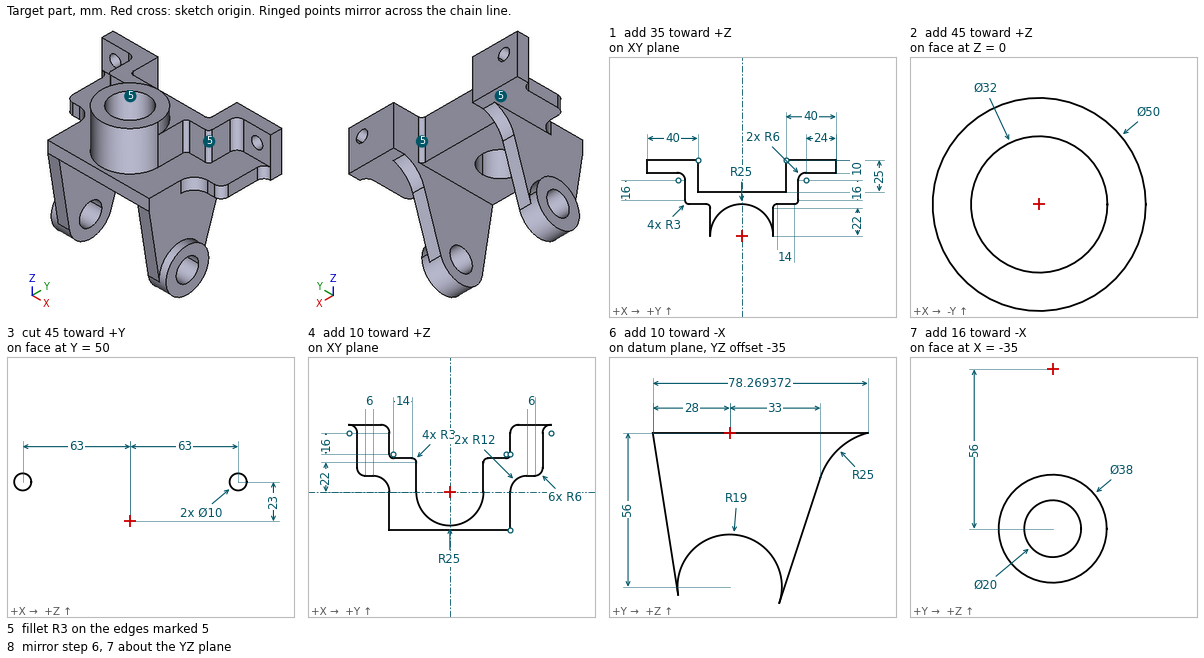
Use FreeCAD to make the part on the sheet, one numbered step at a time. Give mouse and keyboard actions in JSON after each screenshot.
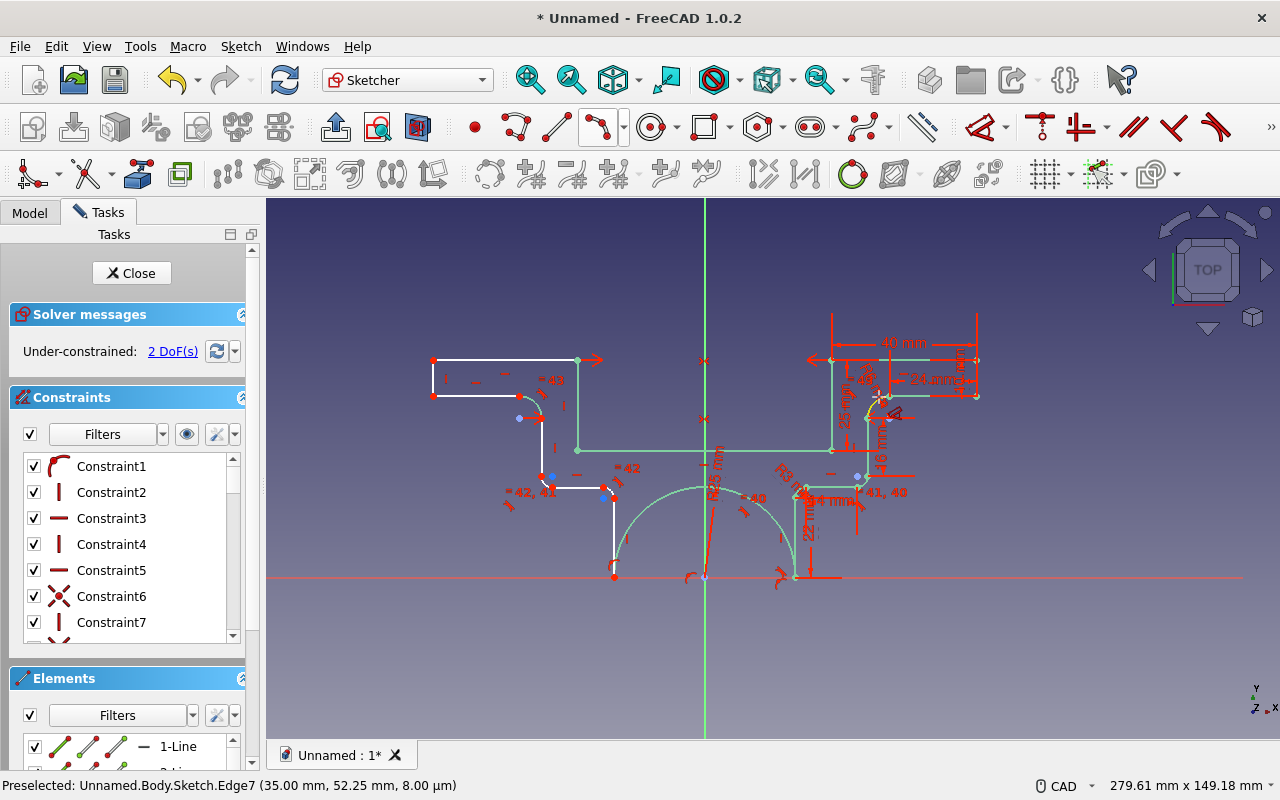
{"action": "left_click", "coordinate": [534, 360]}
{"action": "left_click", "coordinate": [506, 326]}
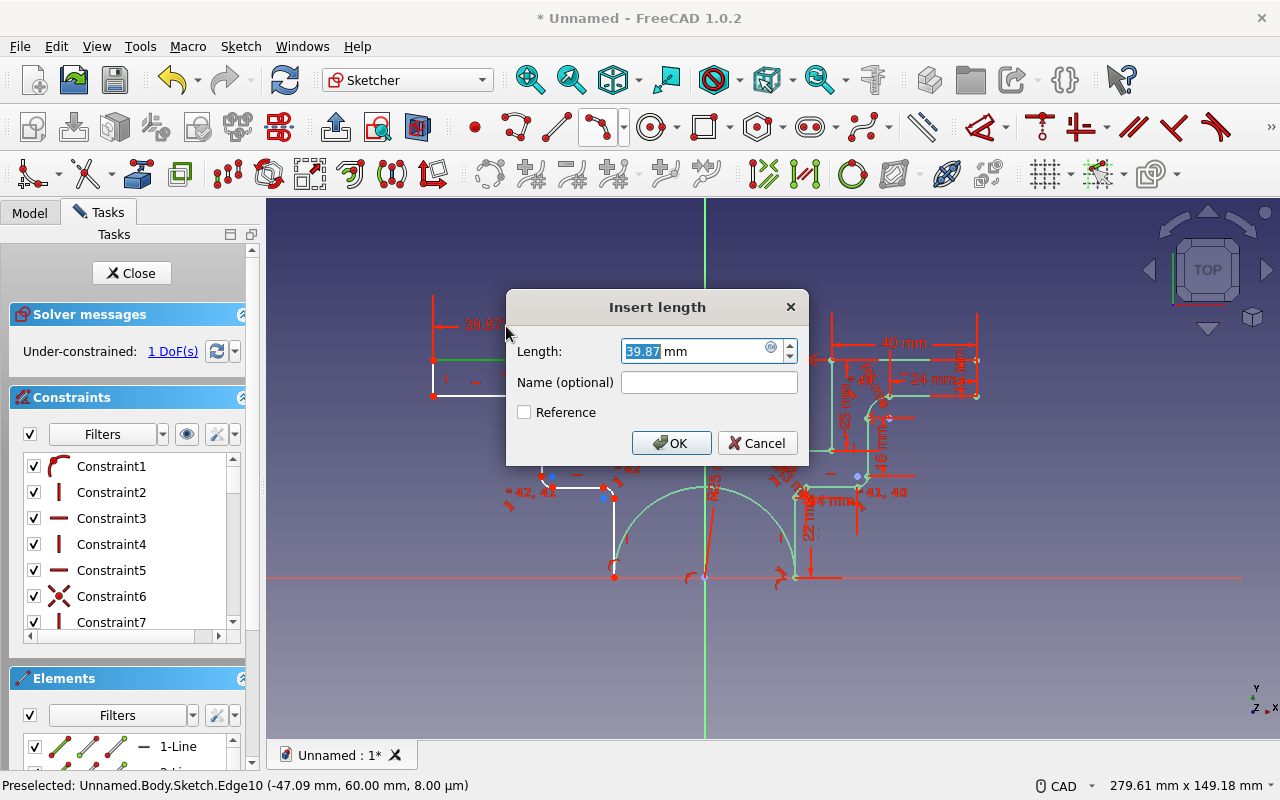
{"action": "type", "text": "40"}
{"action": "key", "text": "Return"}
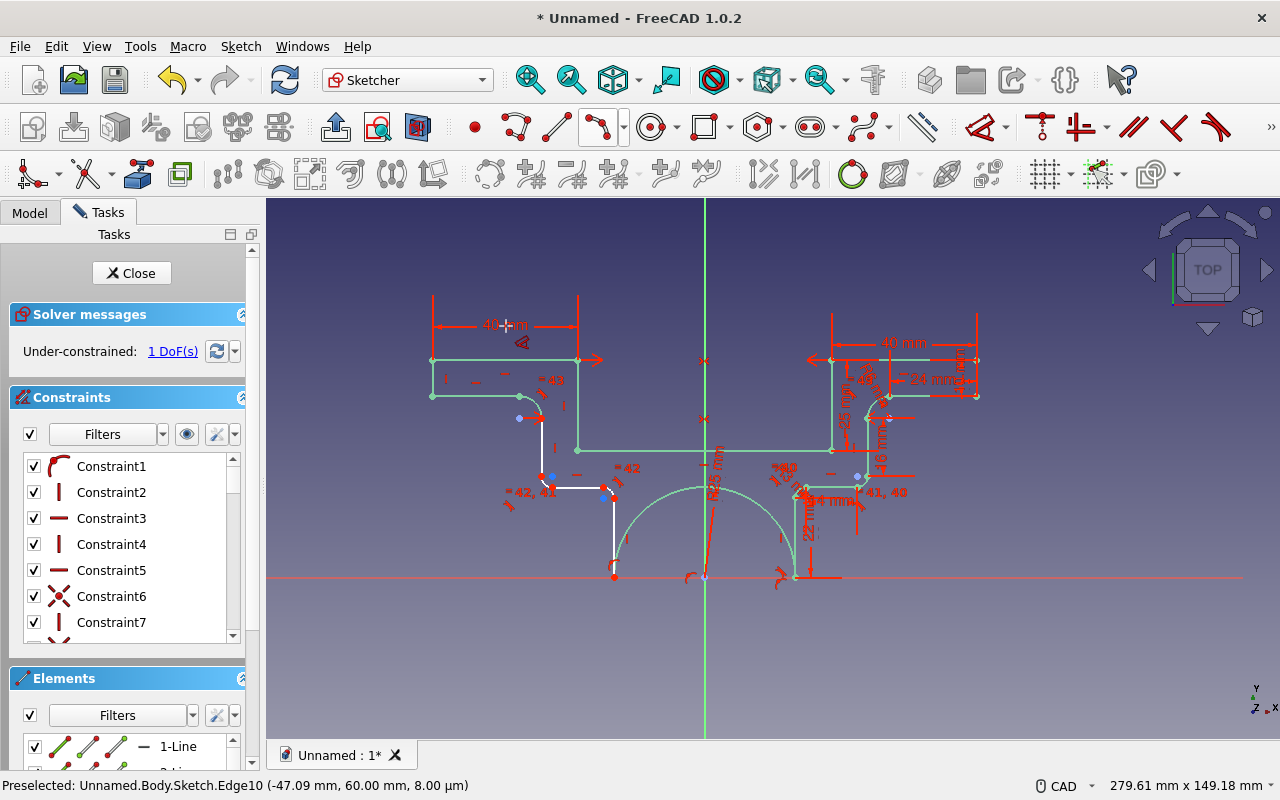
{"action": "left_click", "coordinate": [542, 436]}
{"action": "left_click", "coordinate": [508, 447]}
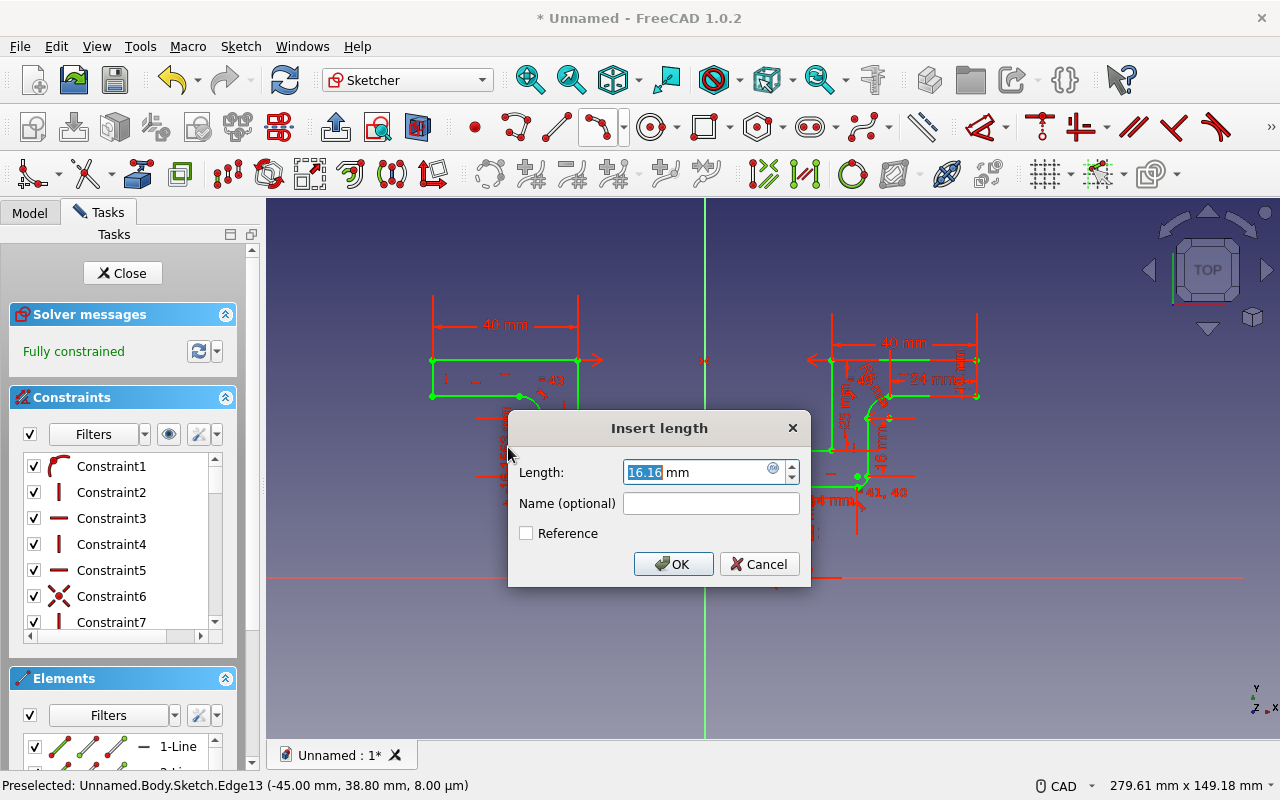
{"action": "type", "text": "16"}
{"action": "key", "text": "Return"}
{"action": "key", "text": "Escape"}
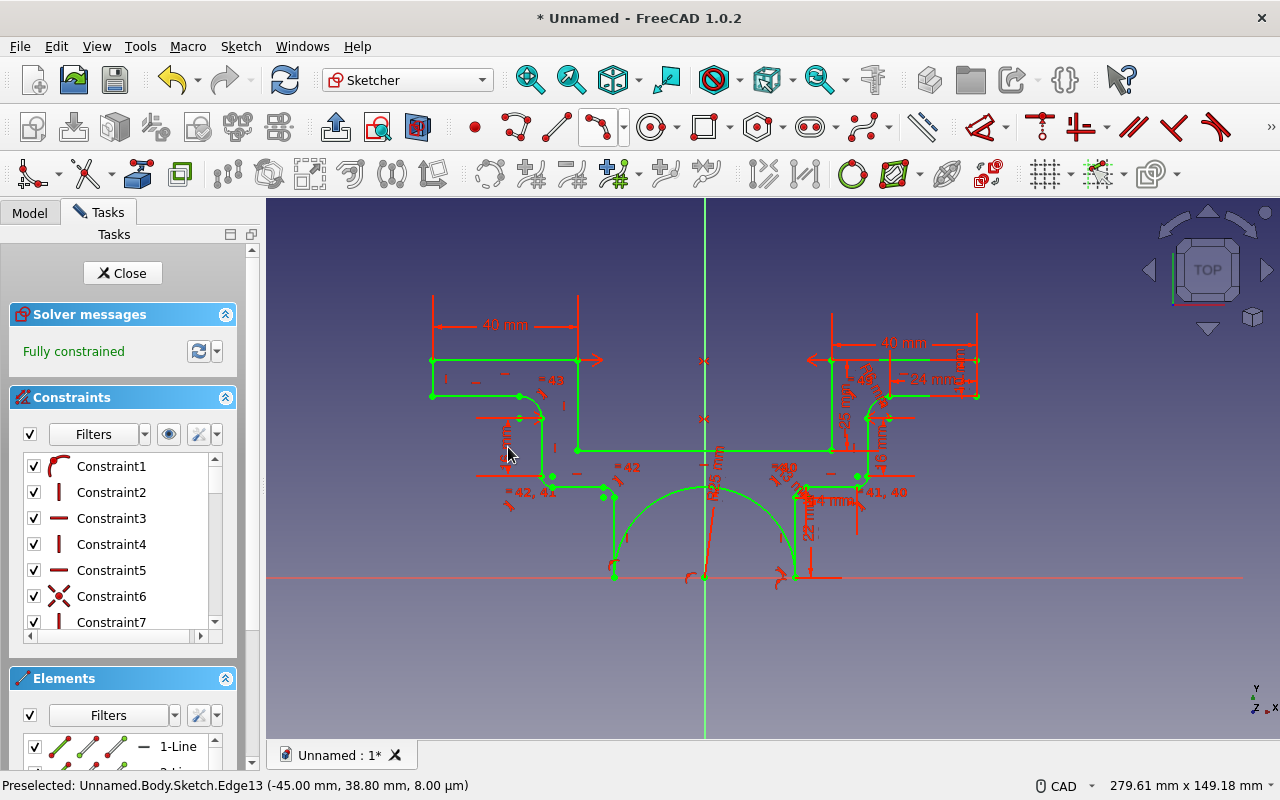
{"action": "left_click", "coordinate": [123, 273]}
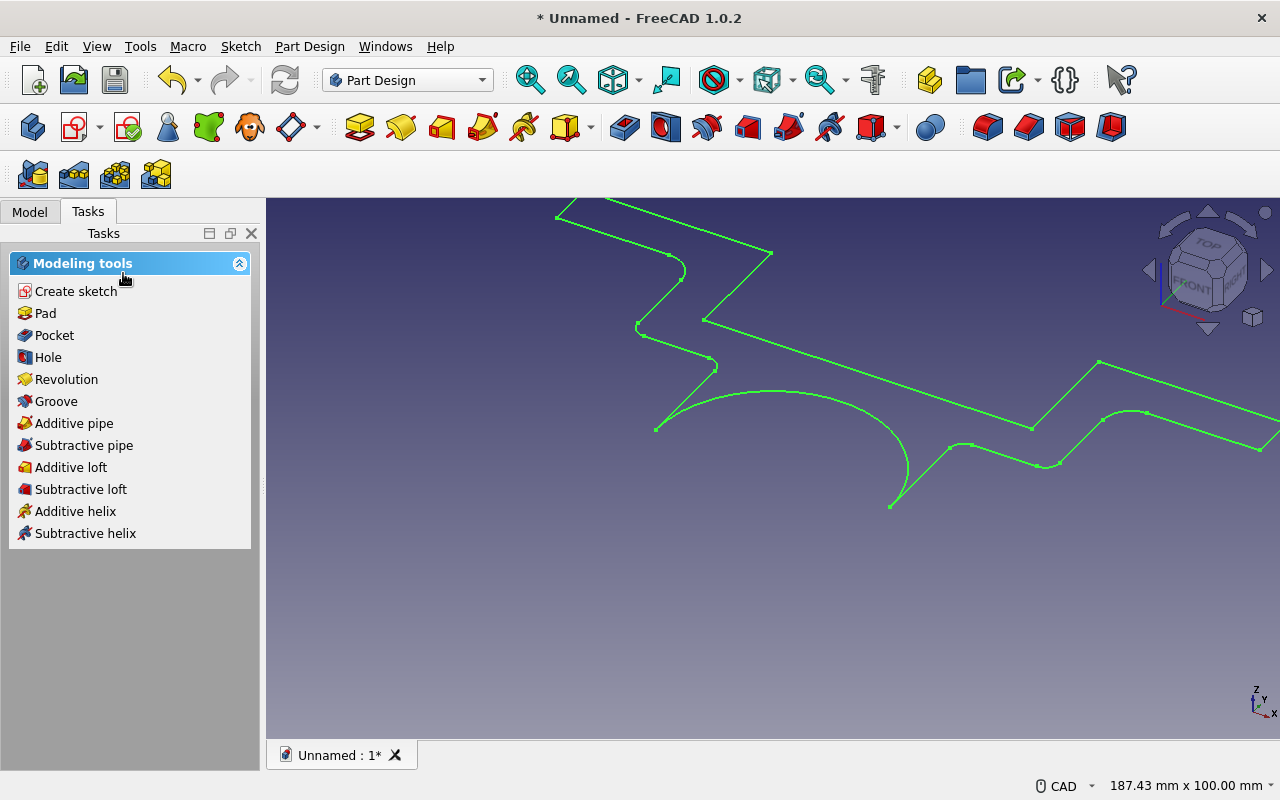
{"action": "left_click", "coordinate": [360, 128]}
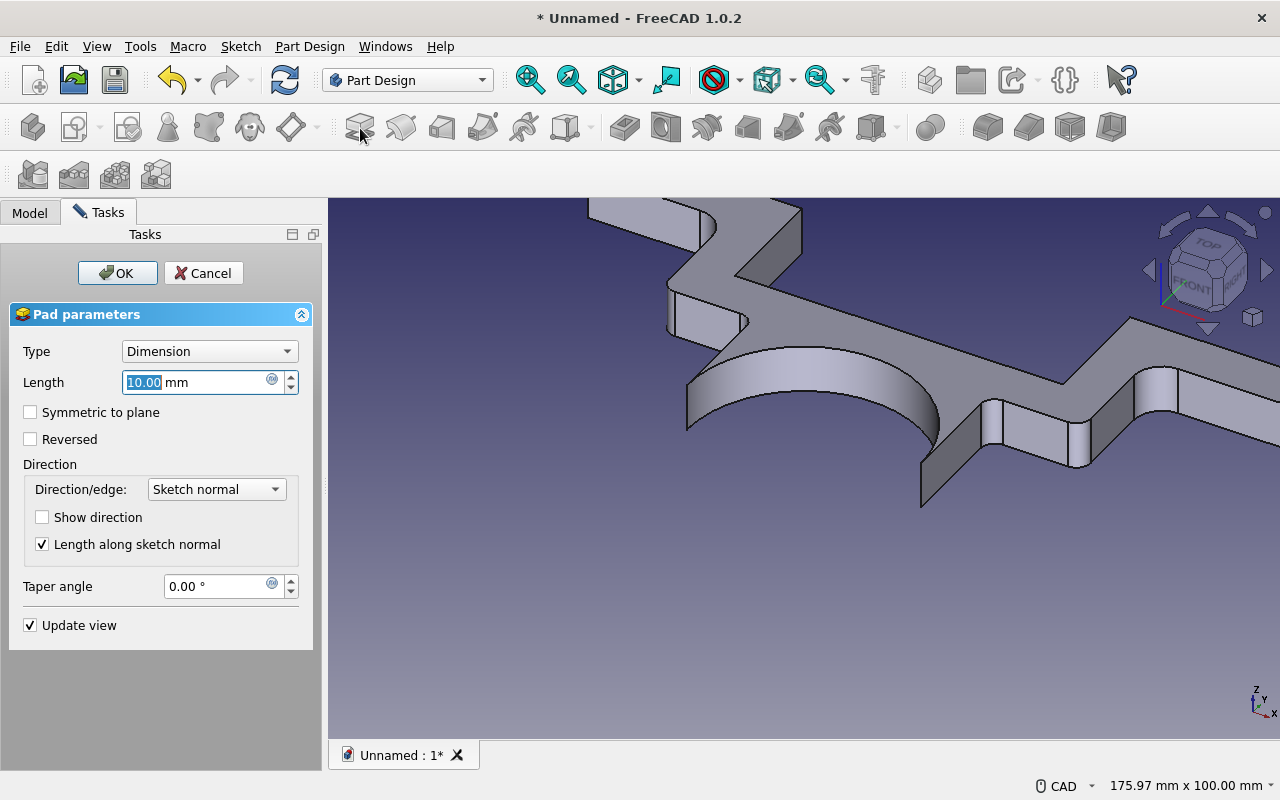
{"action": "type", "text": "35"}
{"action": "key", "text": "Tab"}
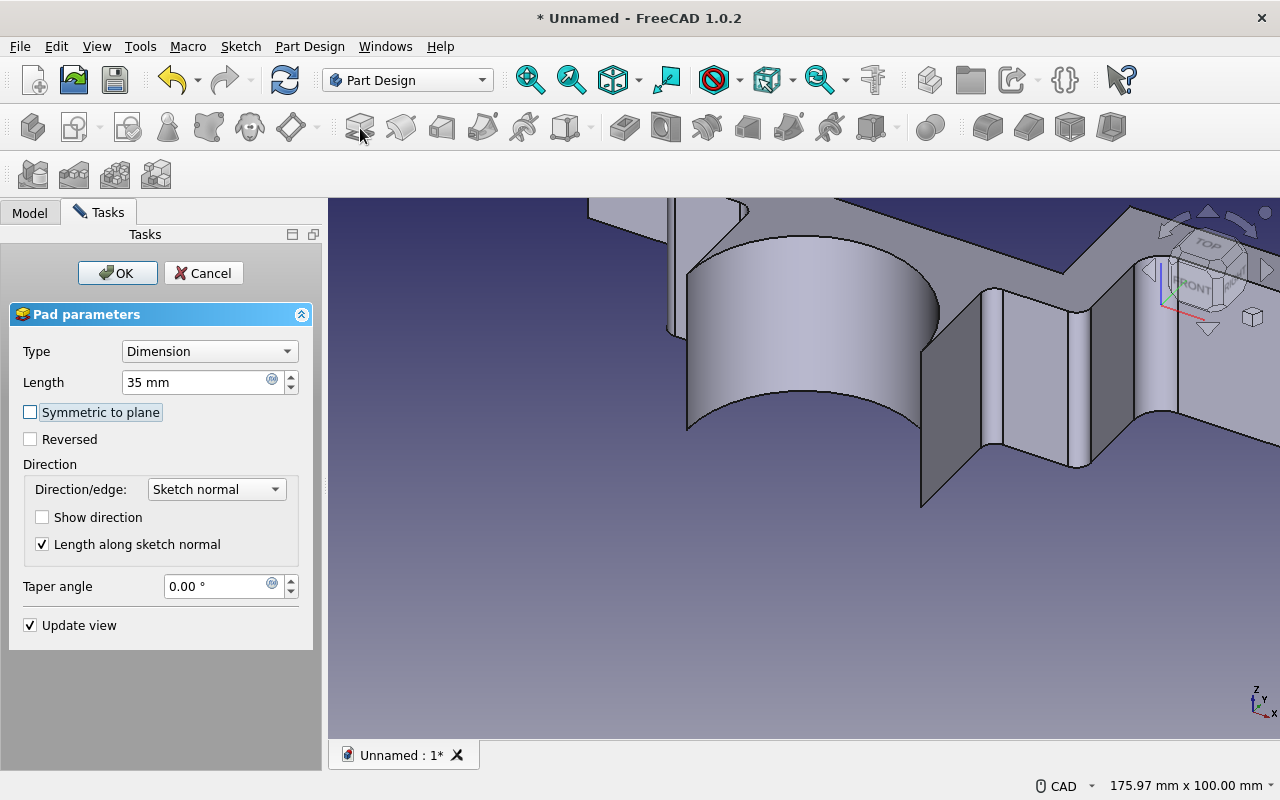
{"action": "left_click", "coordinate": [118, 273]}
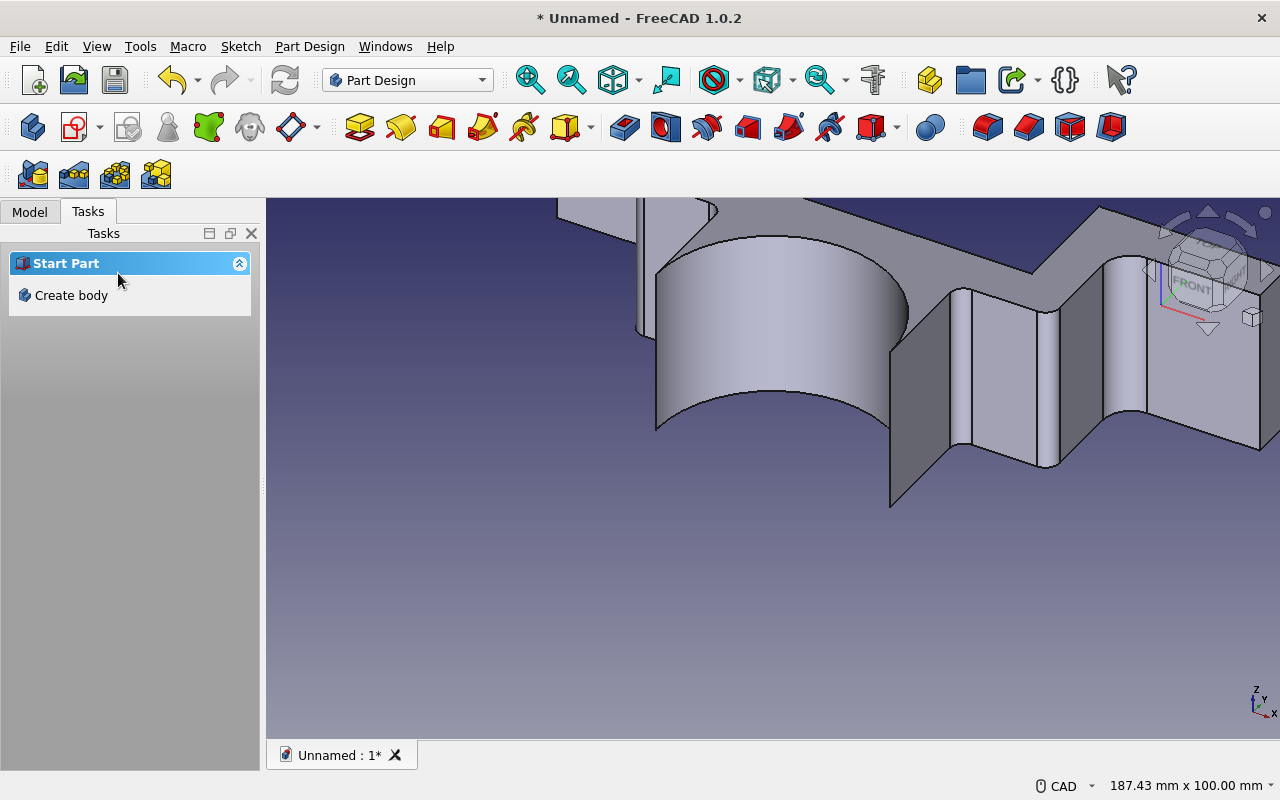
{"action": "left_click", "coordinate": [531, 80]}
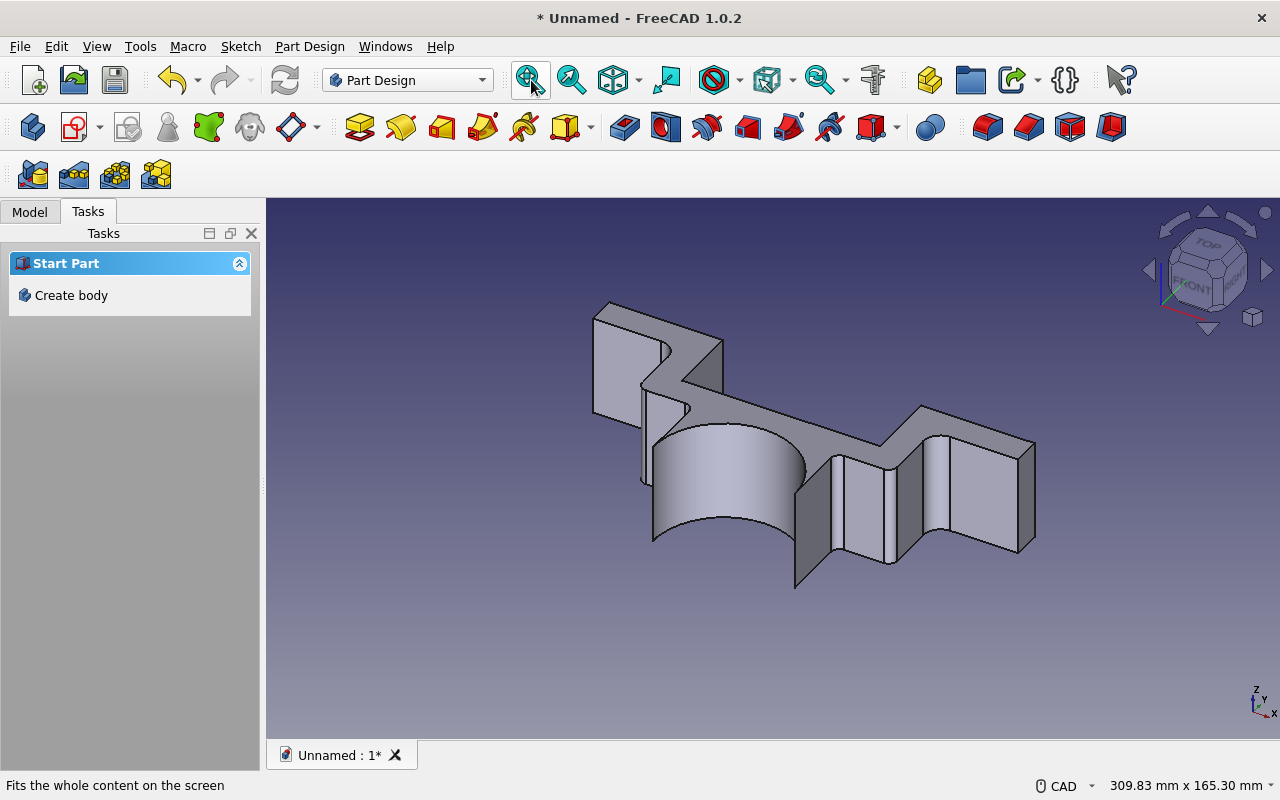
{"action": "key", "text": "5"}